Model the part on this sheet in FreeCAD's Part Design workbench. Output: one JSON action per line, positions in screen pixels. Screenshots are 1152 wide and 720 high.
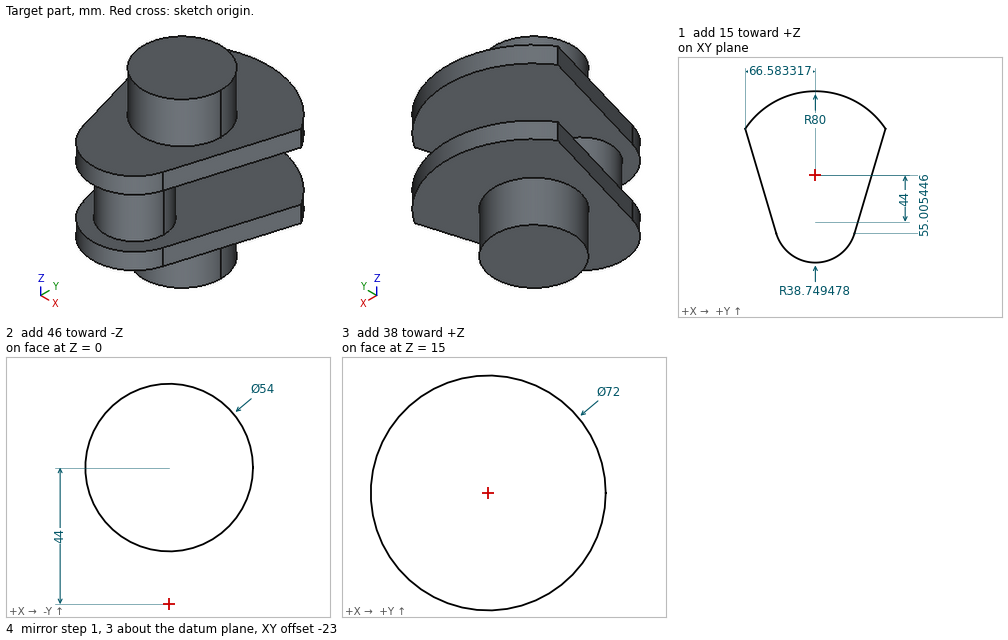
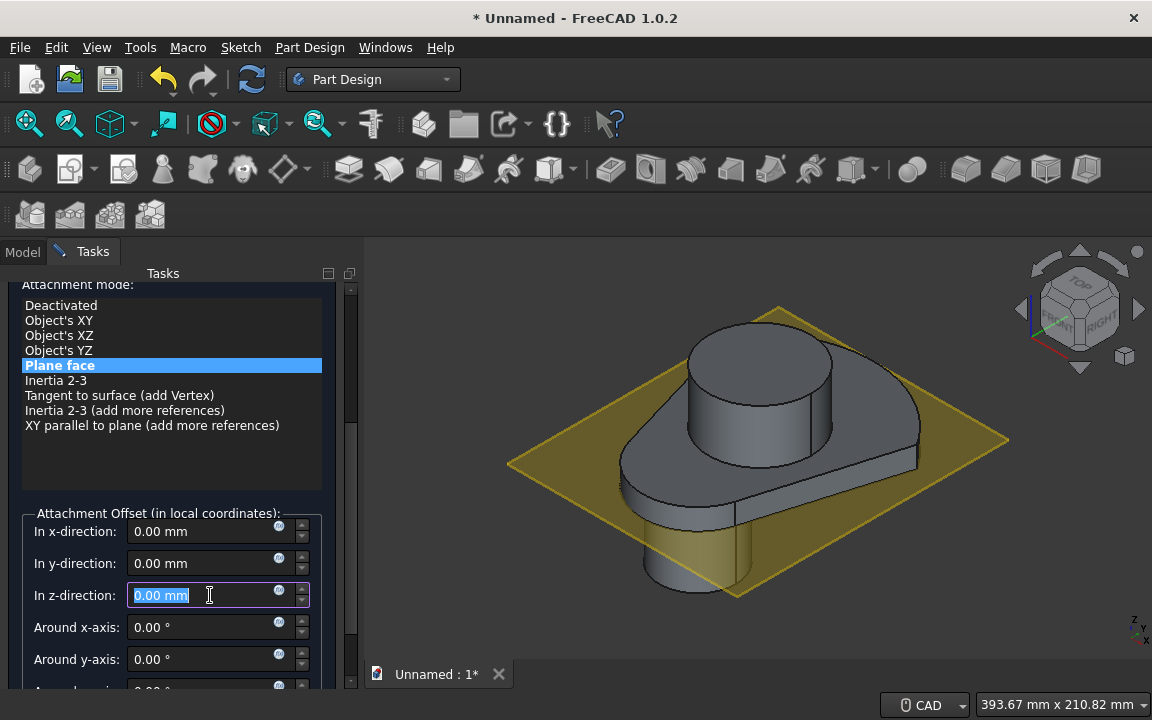
{"action": "type", "text": "-23"}
{"action": "key", "text": "Tab"}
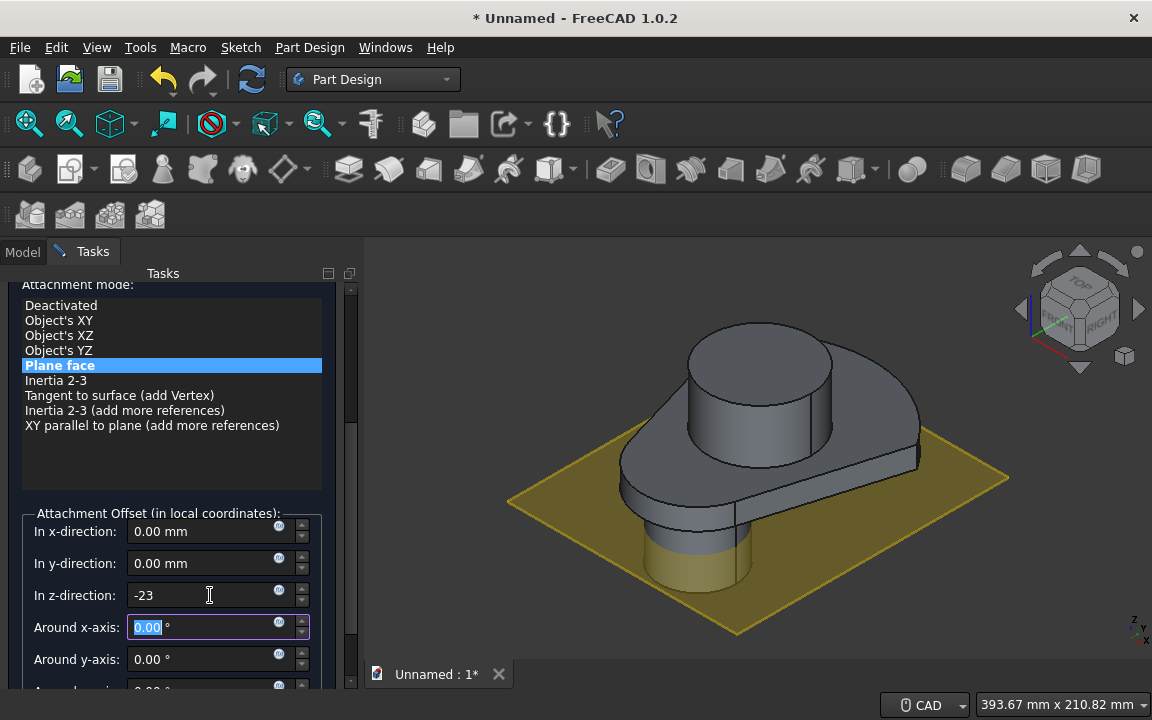
{"action": "scroll", "coordinate": [351, 486], "scroll_direction": "up", "scroll_amount": 5}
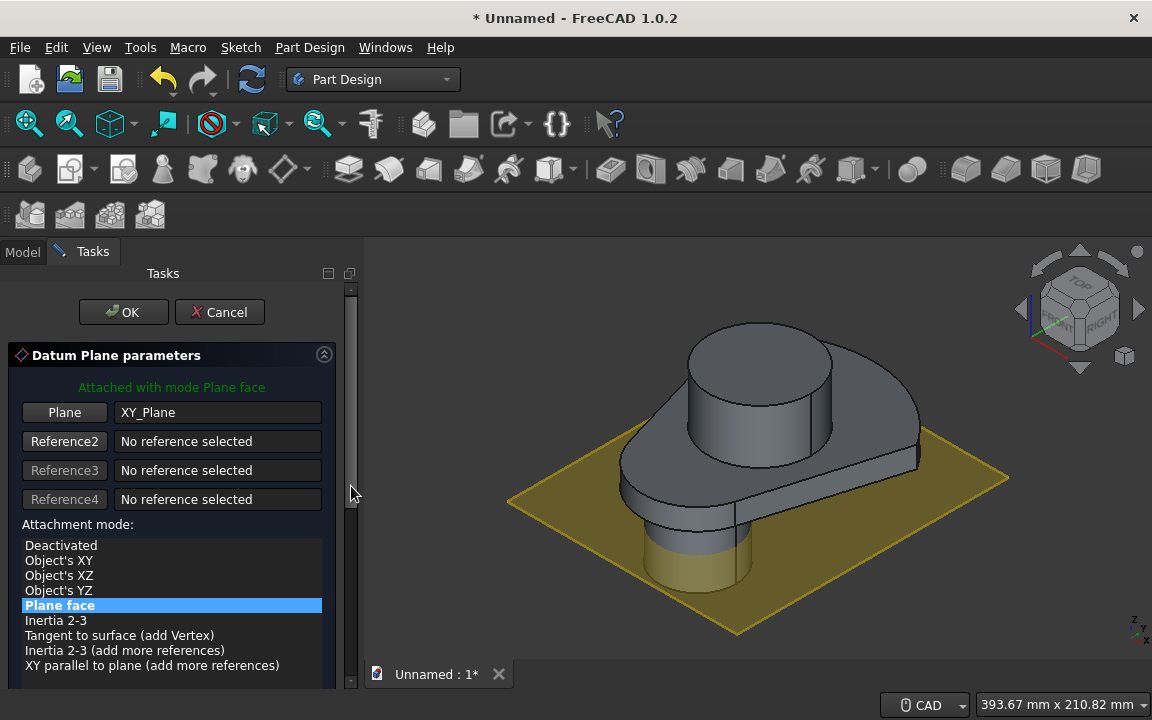
{"action": "left_click", "coordinate": [124, 312]}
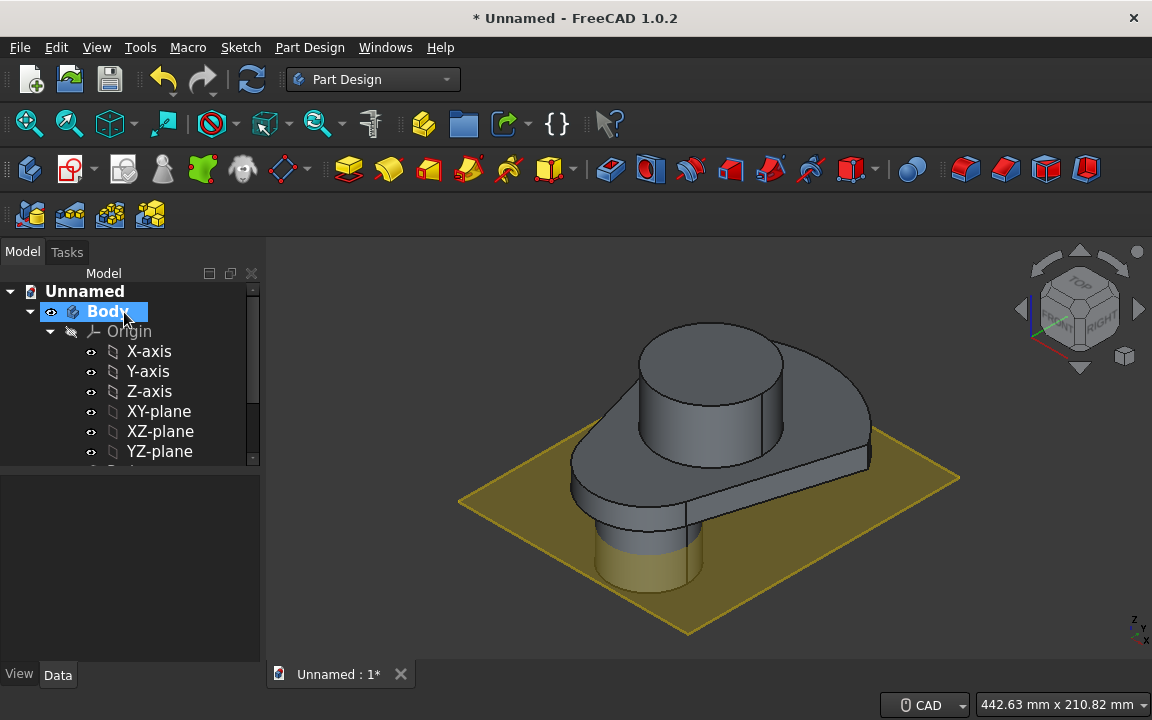
{"action": "scroll", "coordinate": [100, 367], "scroll_direction": "down", "scroll_amount": 3}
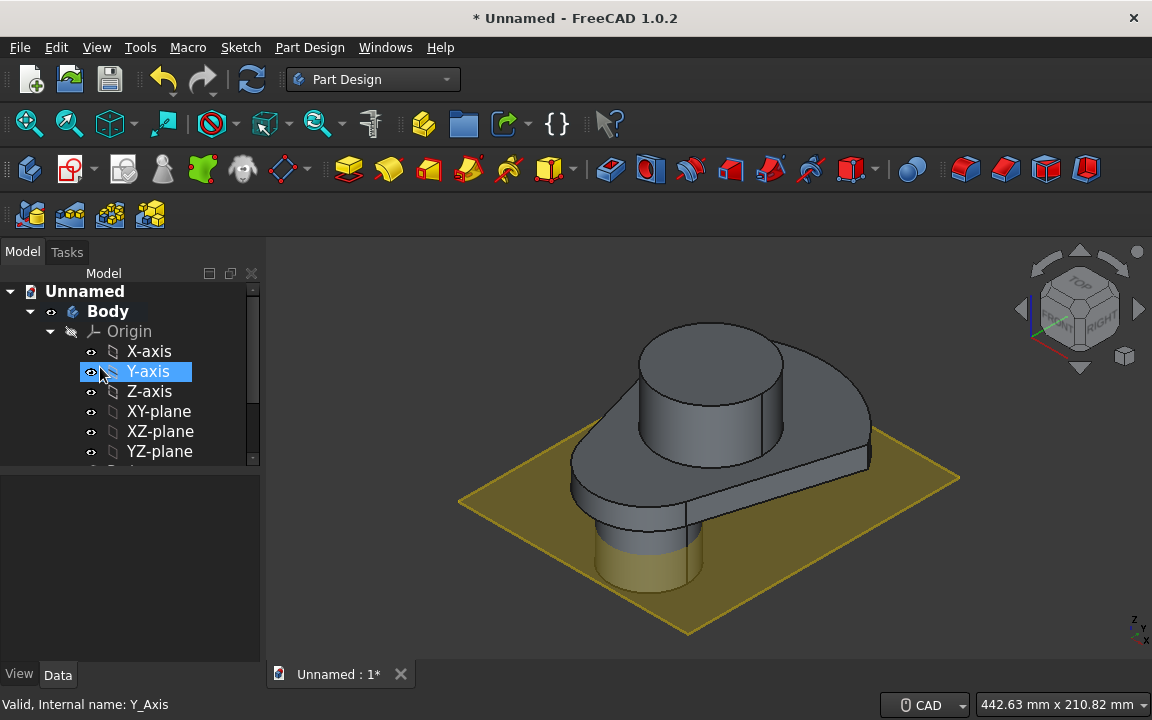
{"action": "left_click", "coordinate": [116, 392]}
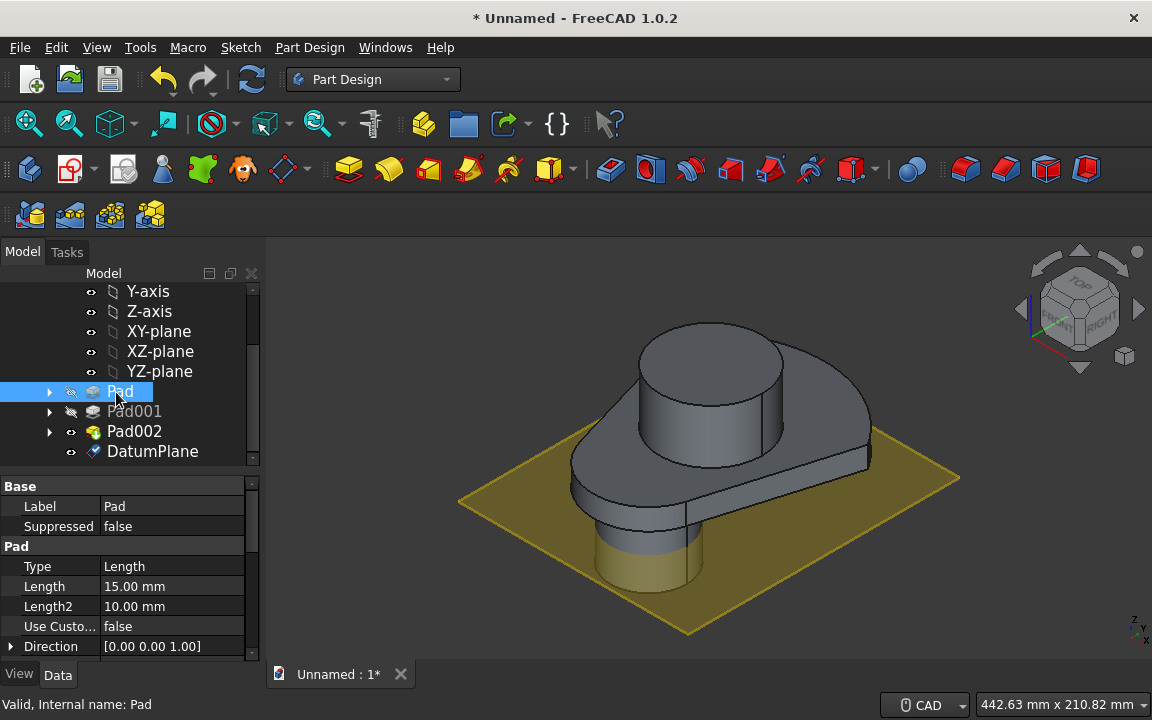
{"action": "left_click", "coordinate": [116, 432], "text": "ctrl"}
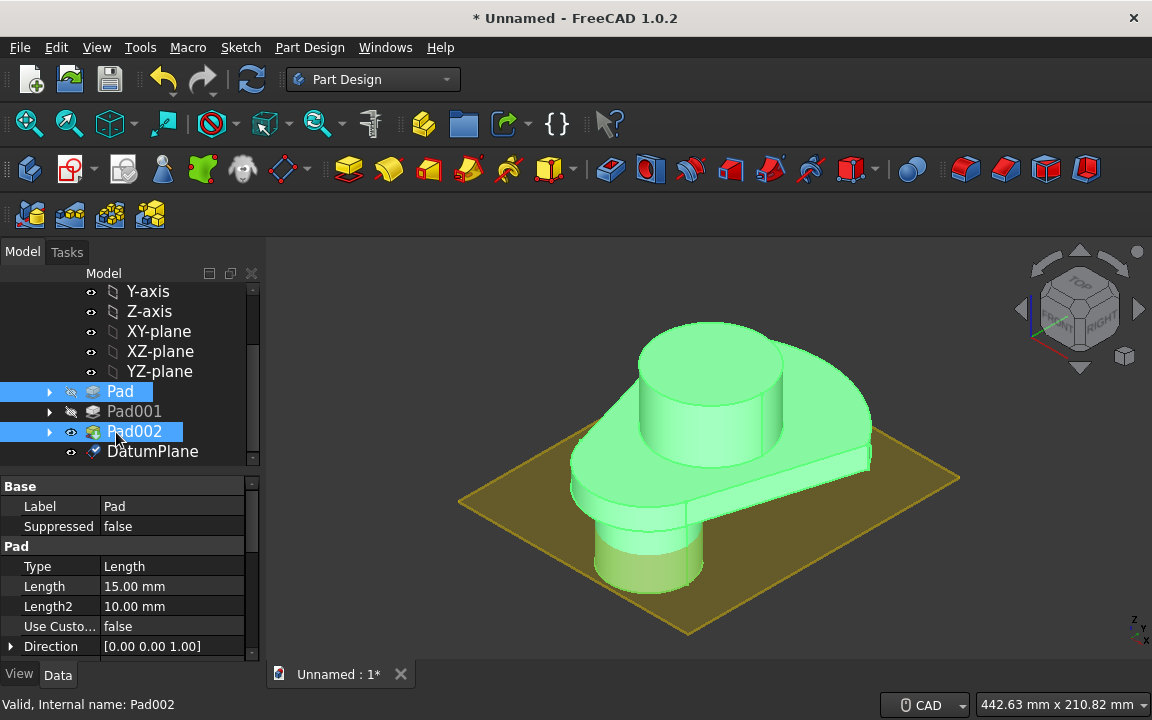
{"action": "left_click", "coordinate": [30, 214]}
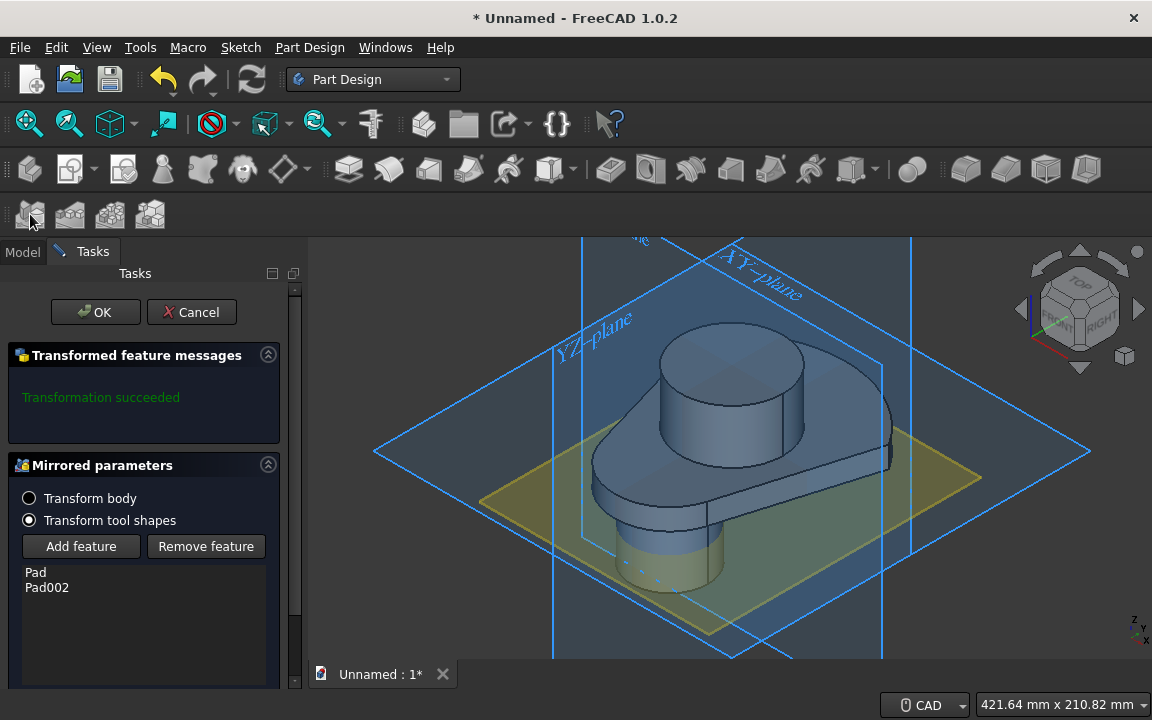
{"action": "scroll", "coordinate": [295, 486], "scroll_direction": "down", "scroll_amount": 2}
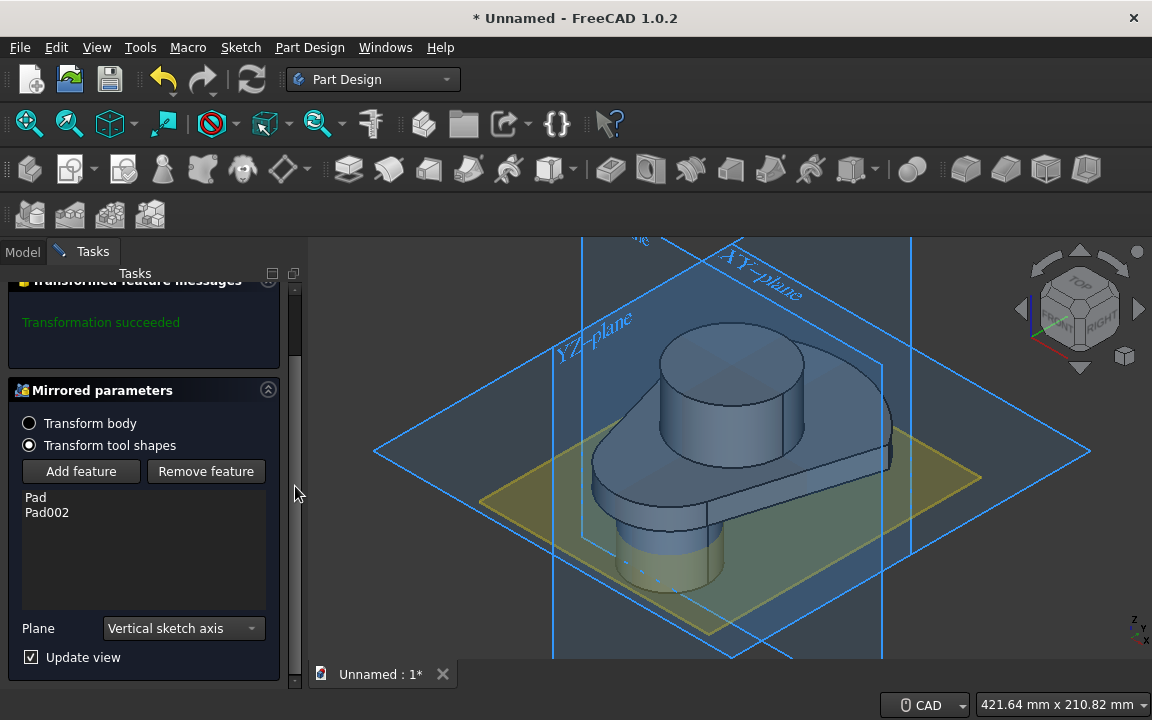
{"action": "left_click", "coordinate": [184, 628]}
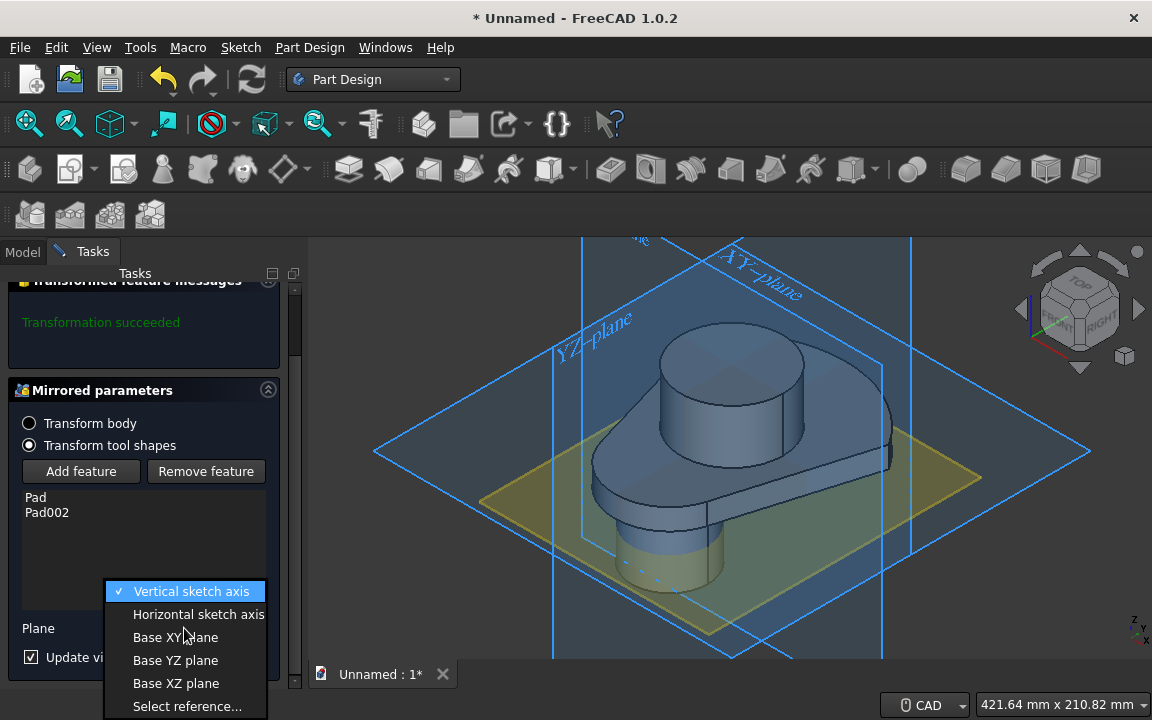
{"action": "left_click", "coordinate": [184, 706]}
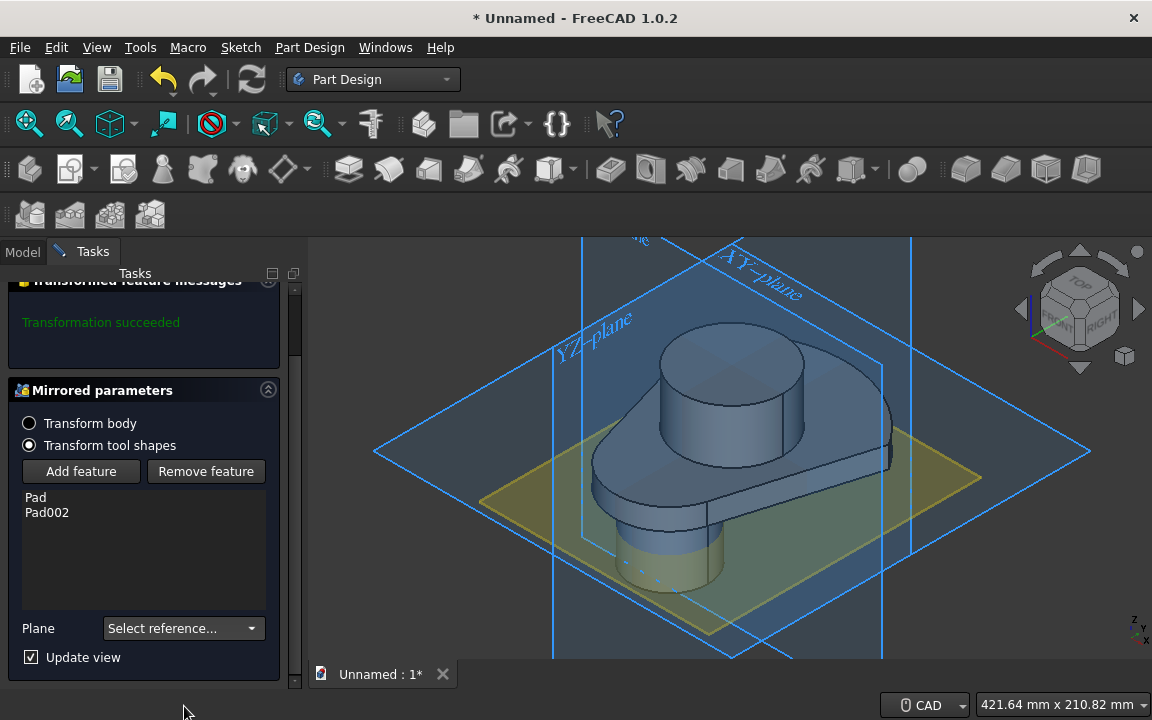
{"action": "left_click", "coordinate": [23, 251]}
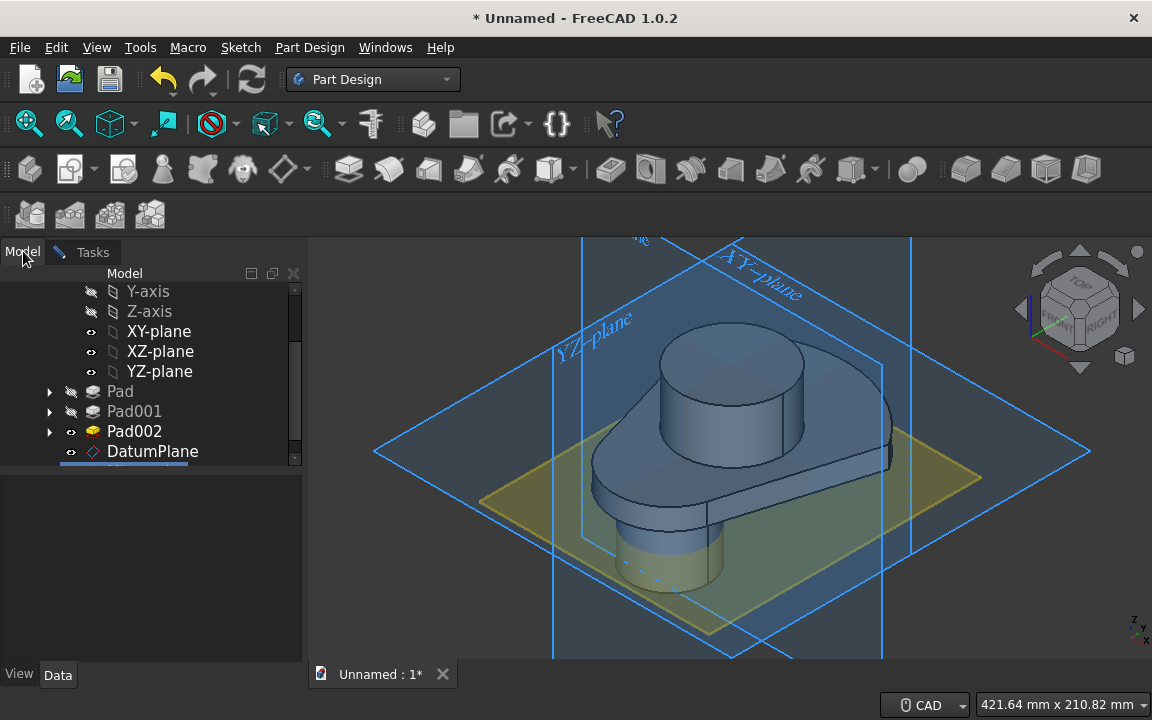
{"action": "left_click", "coordinate": [116, 452]}